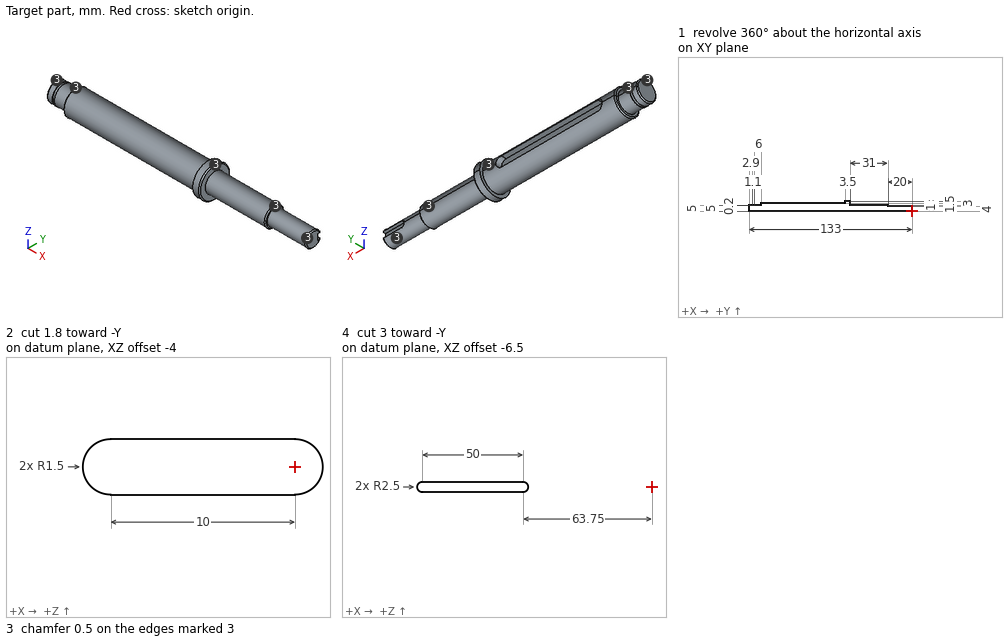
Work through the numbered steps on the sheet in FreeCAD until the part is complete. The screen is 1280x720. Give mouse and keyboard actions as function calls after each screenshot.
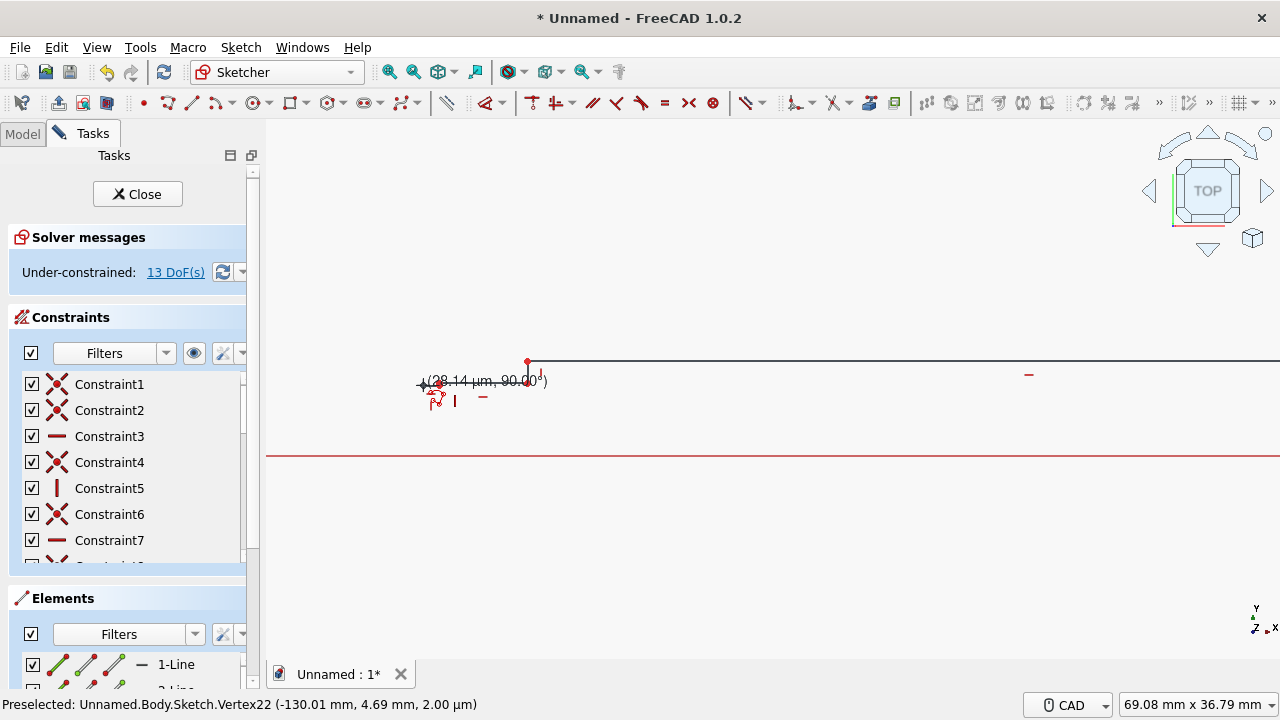
scroll(423, 382, up, 9)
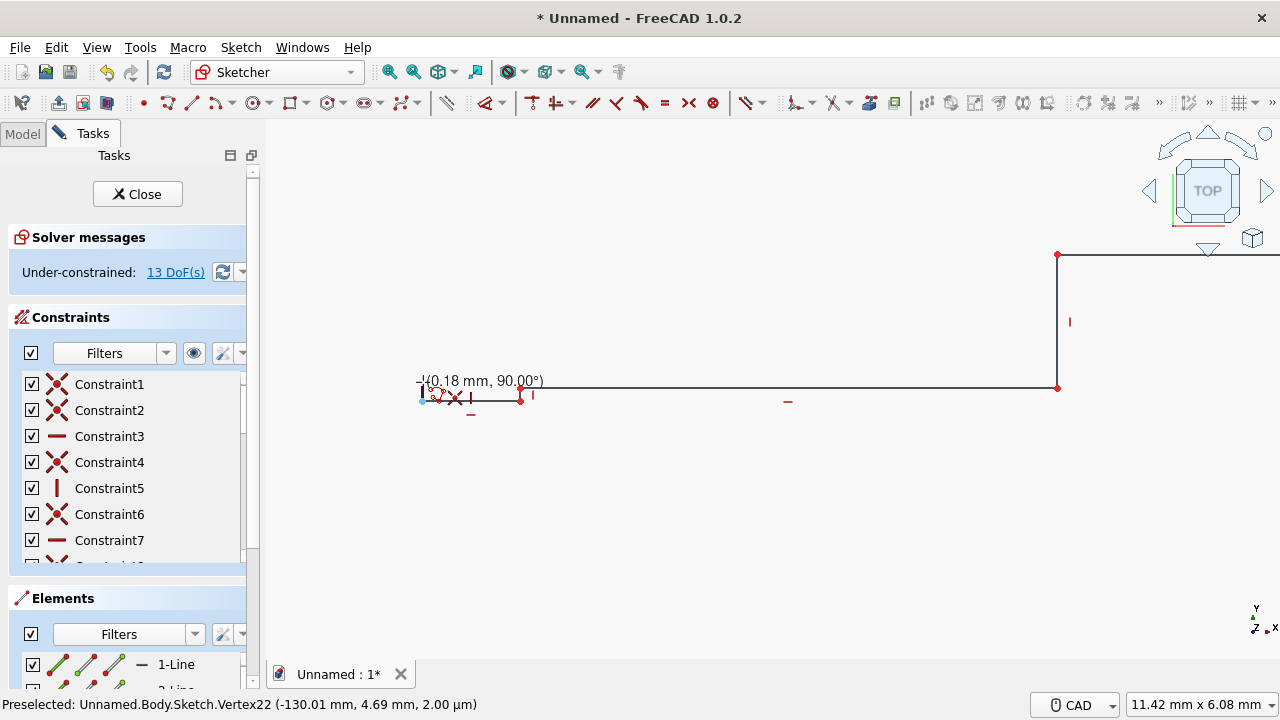
click(422, 382)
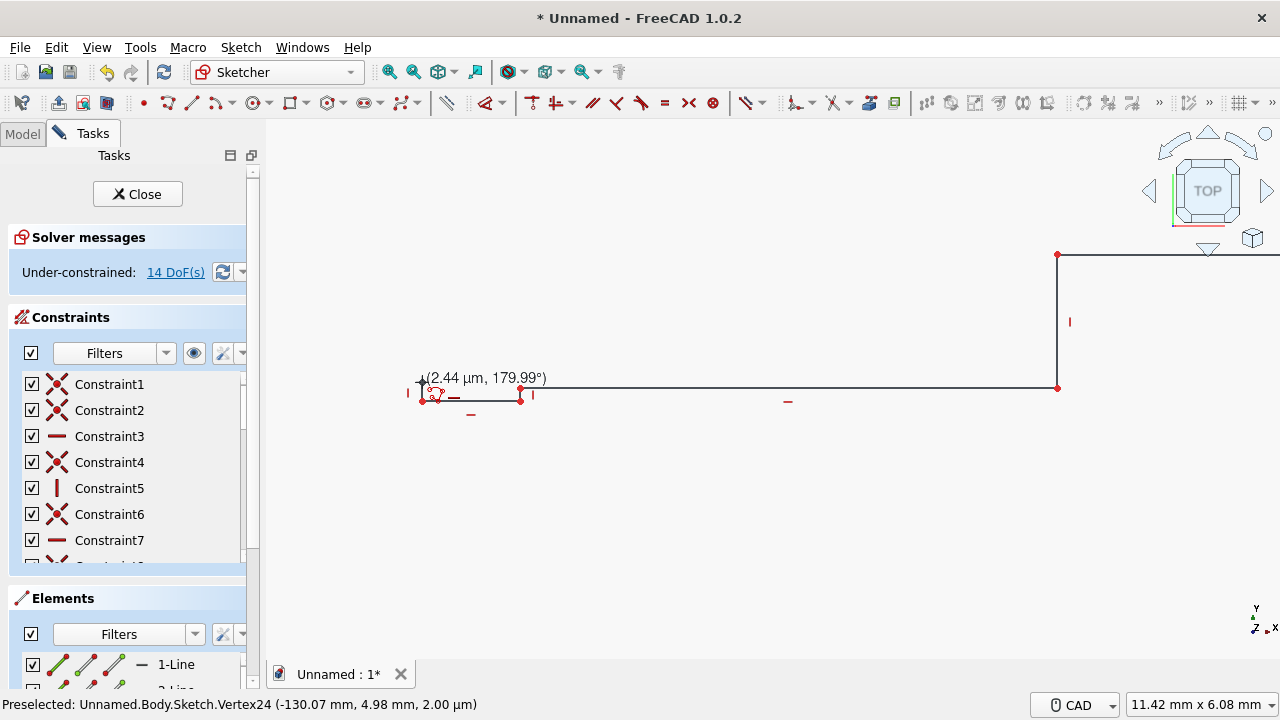
scroll(423, 385, down, 15)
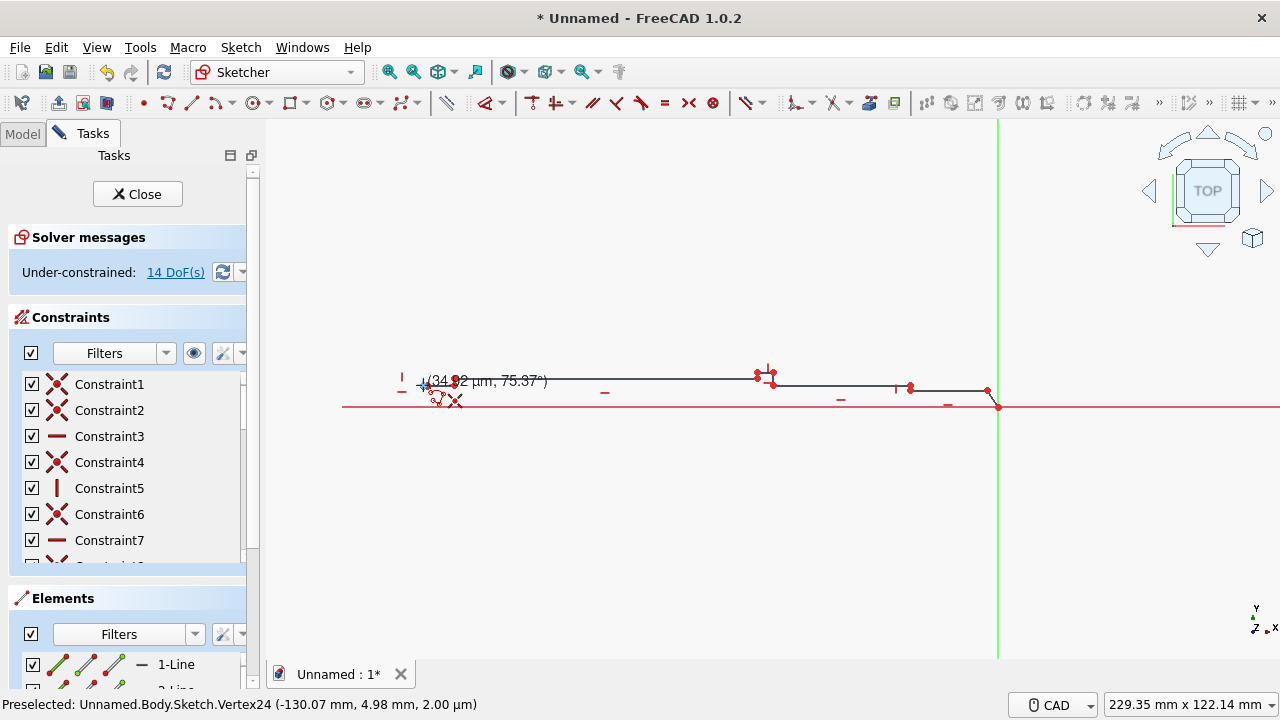
scroll(410, 385, up, 2)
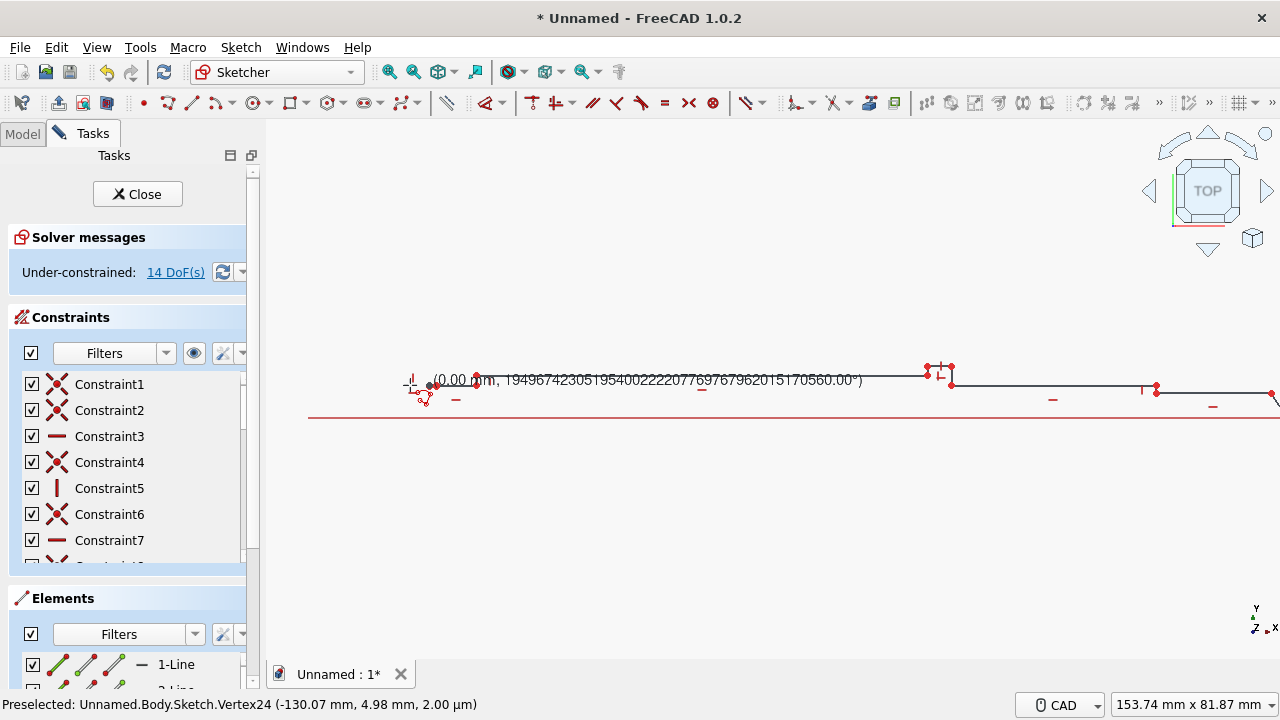
click(410, 385)
click(410, 409)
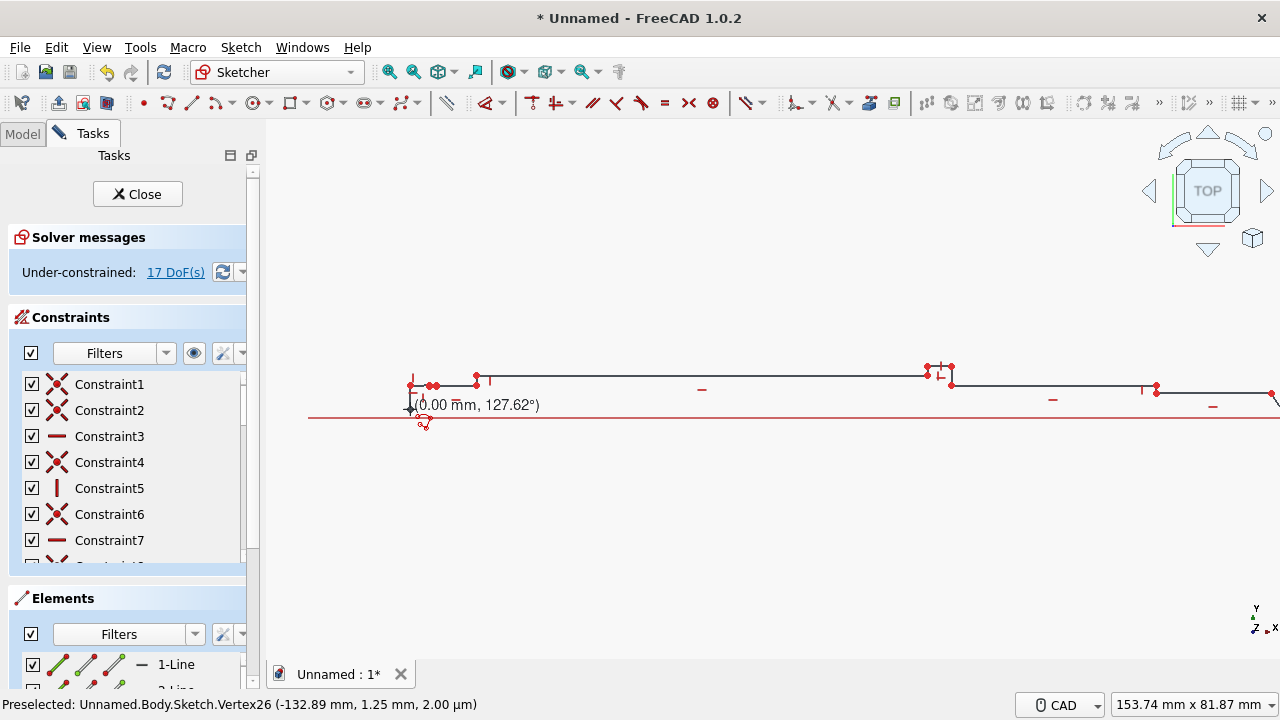
scroll(411, 383, down, 2)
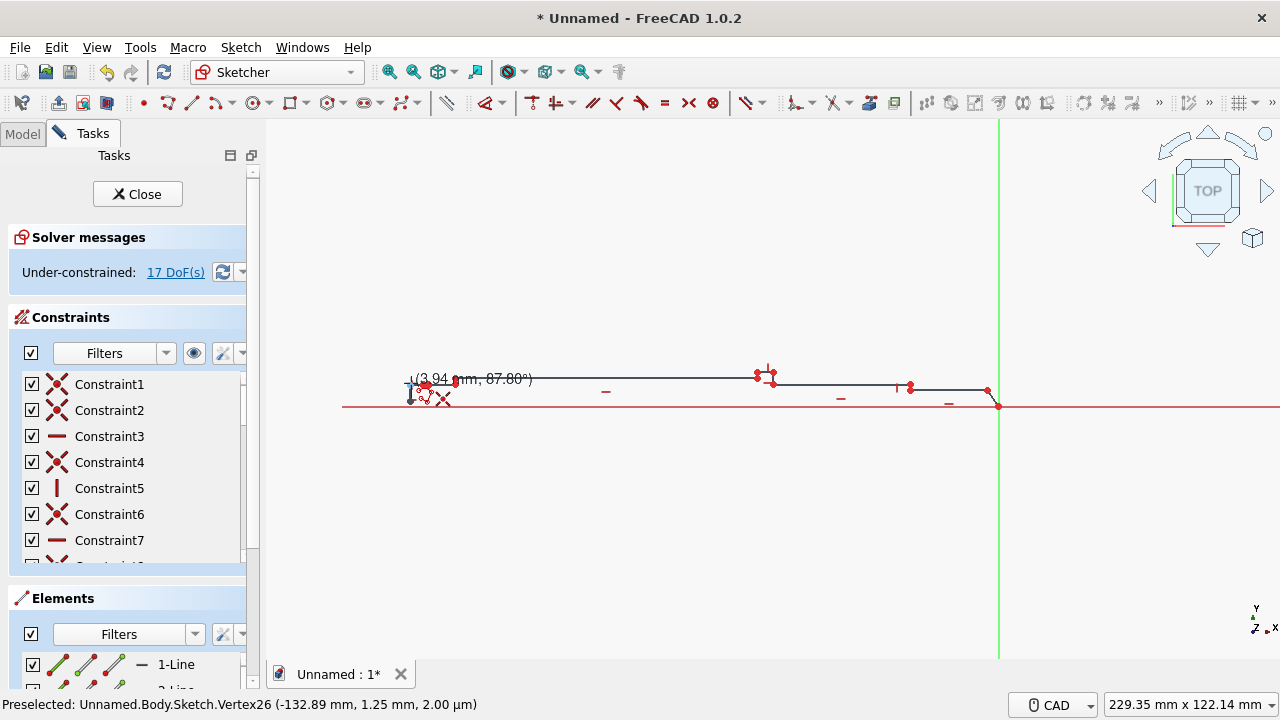
scroll(999, 407, up, 3)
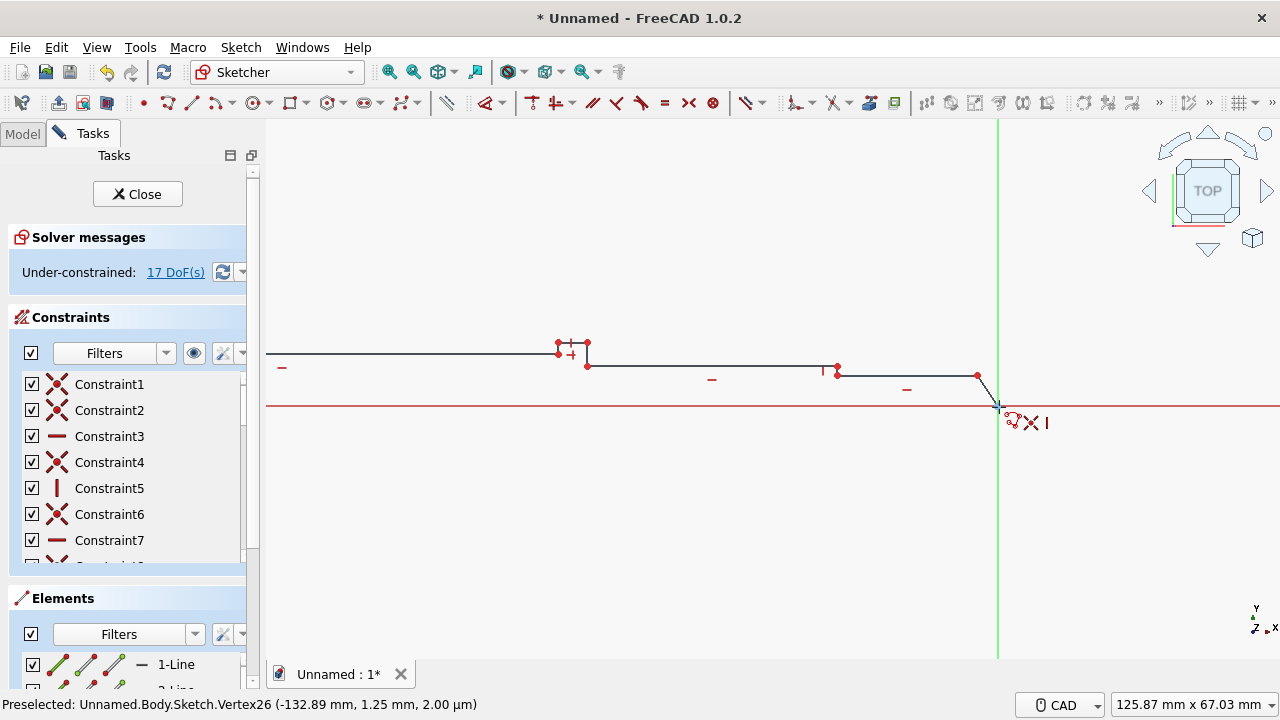
click(998, 406)
key(Escape)
key(Escape)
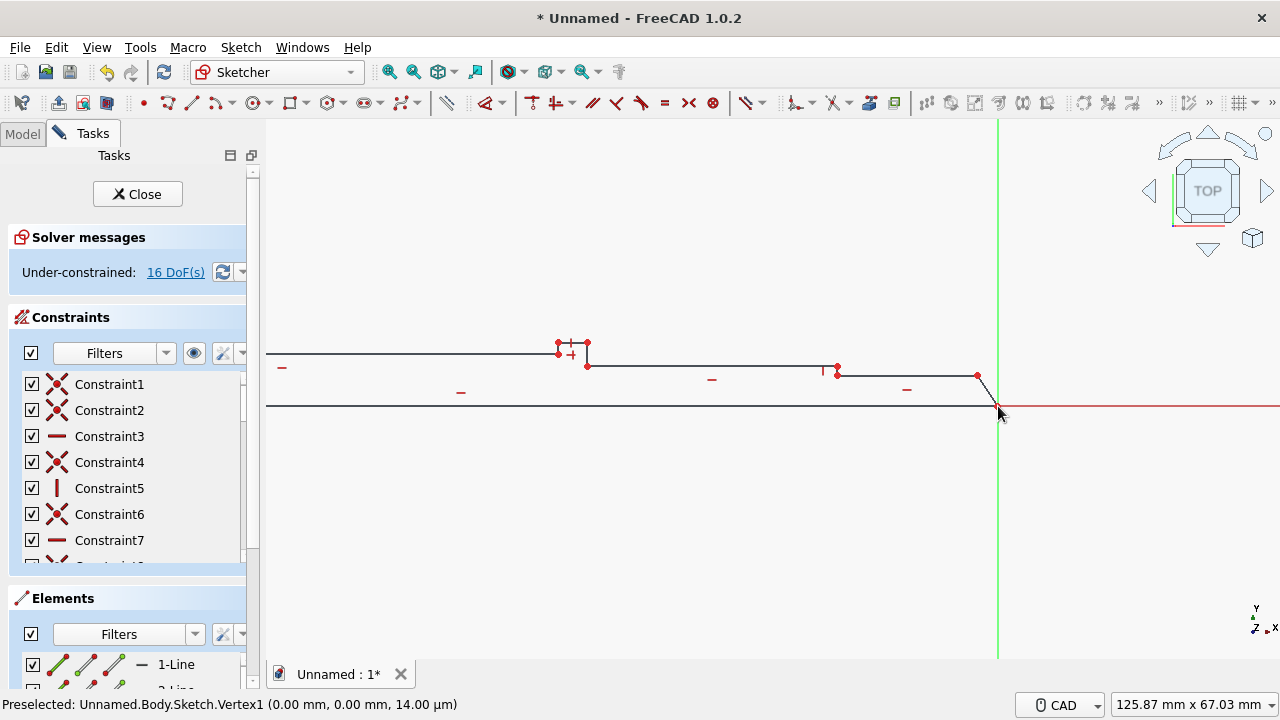
scroll(984, 385, up, 2)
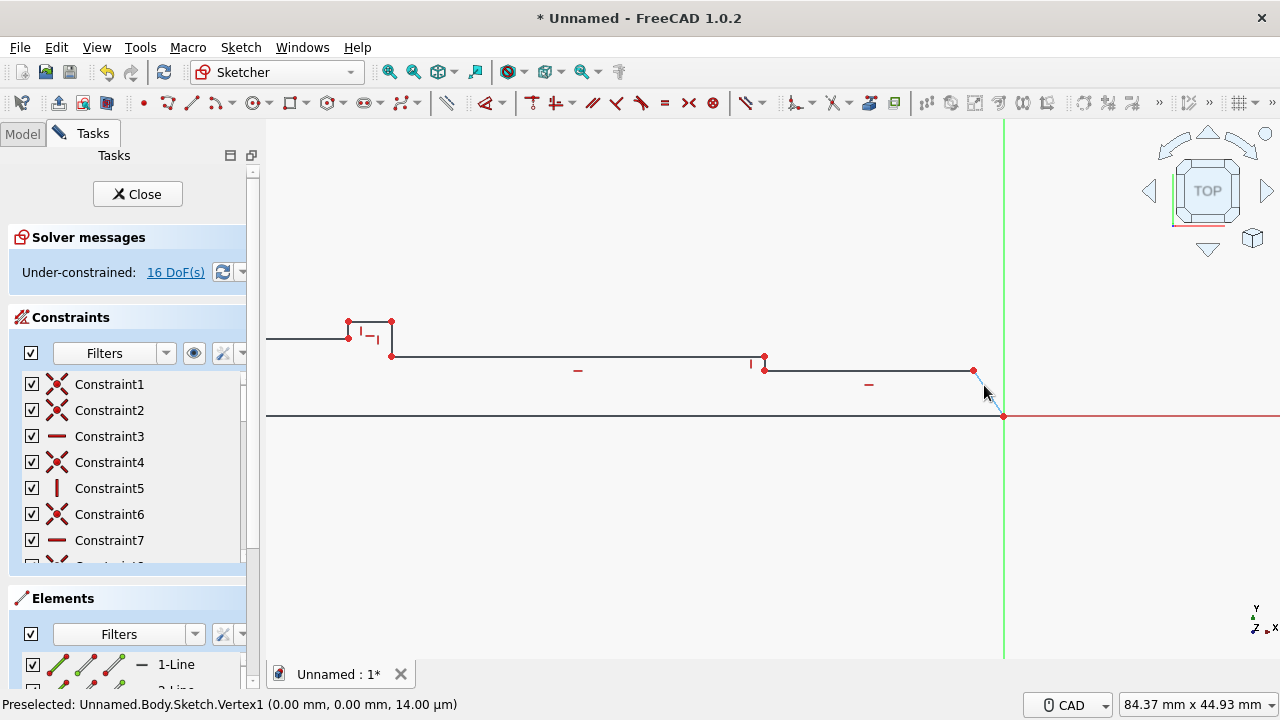
click(983, 384)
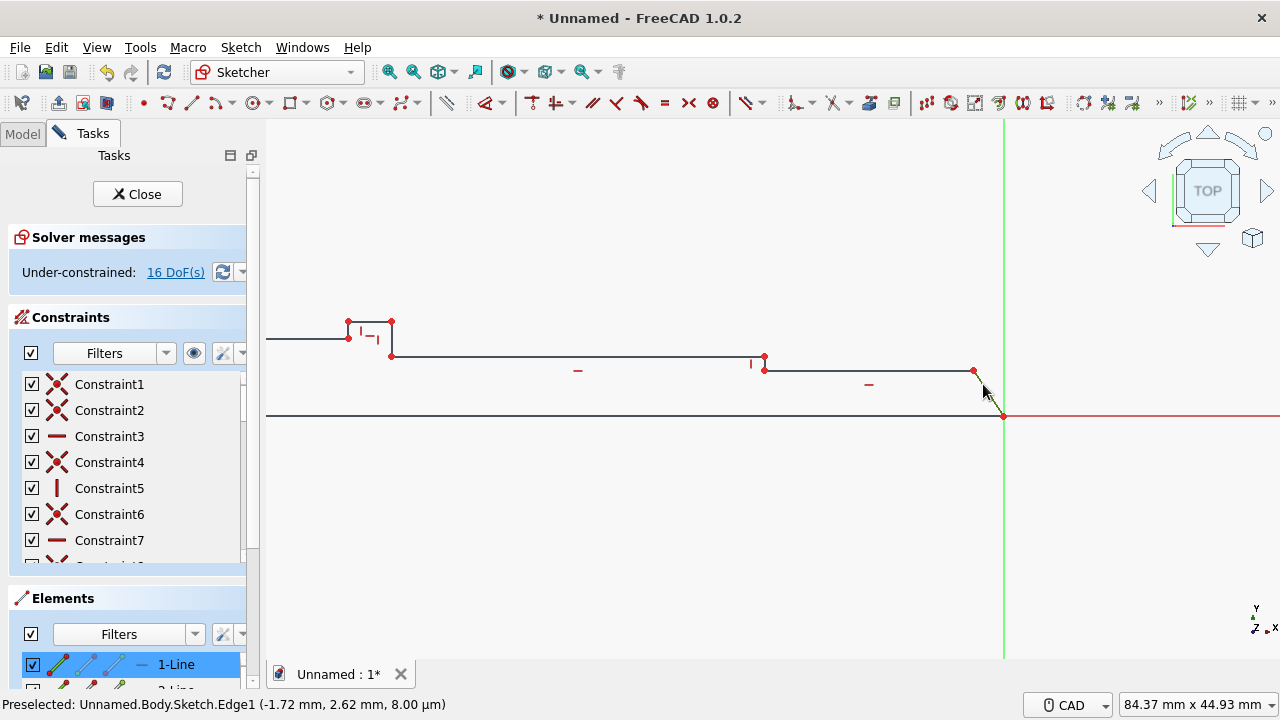
key(v)